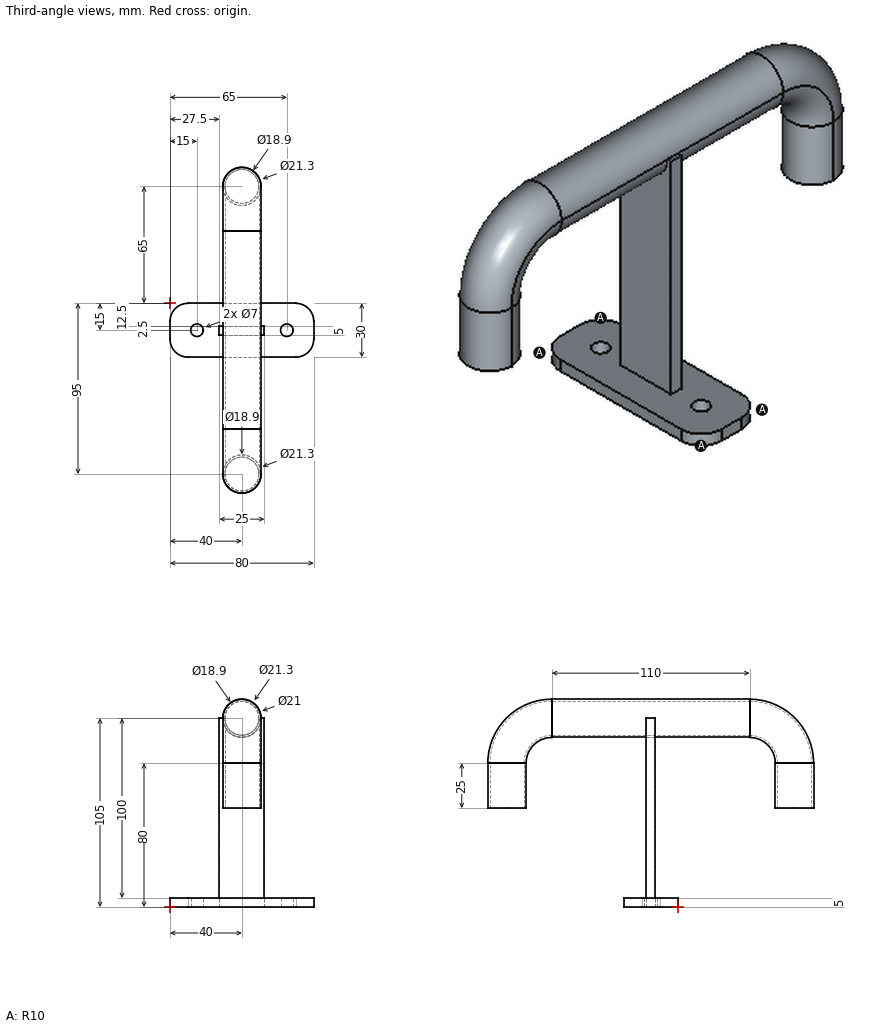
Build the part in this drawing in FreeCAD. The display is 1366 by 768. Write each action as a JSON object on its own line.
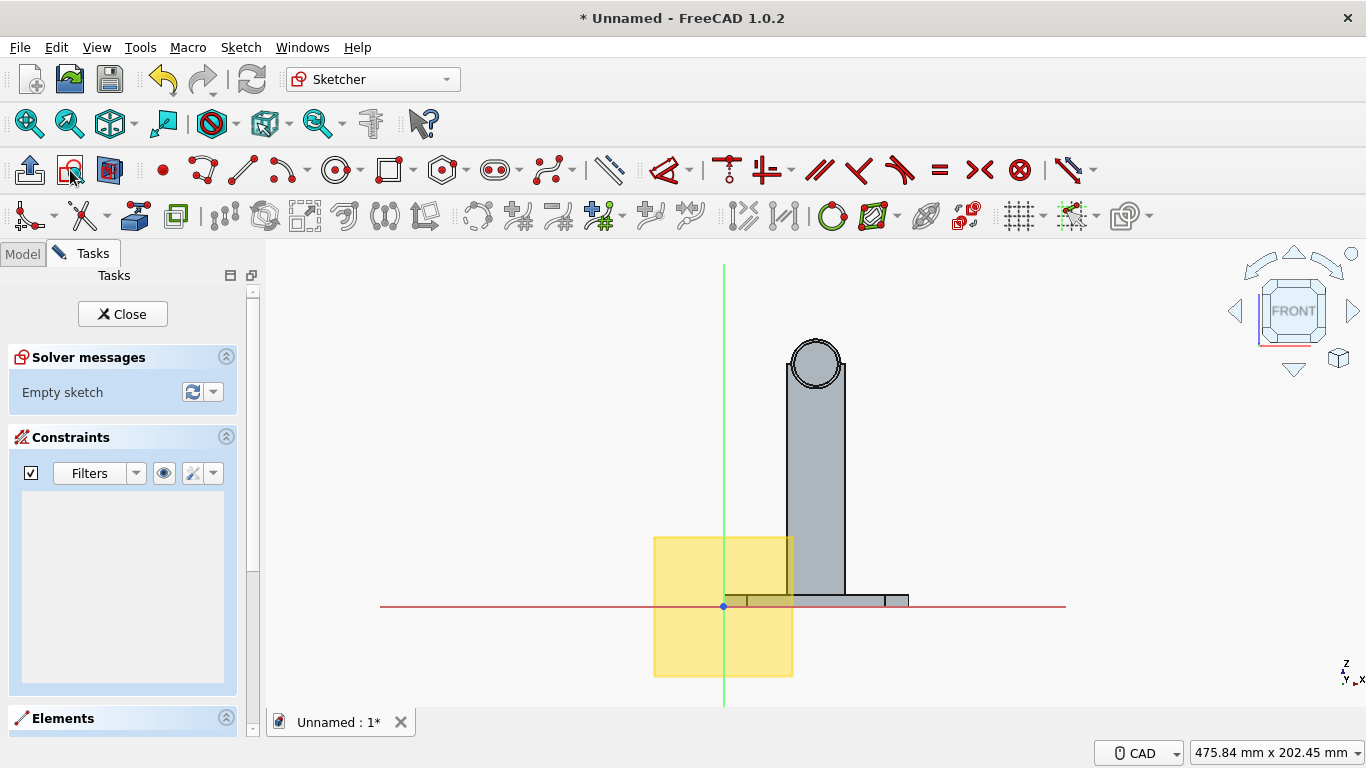
{"action": "scroll", "coordinate": [846, 341], "scroll_direction": "up", "scroll_amount": 6}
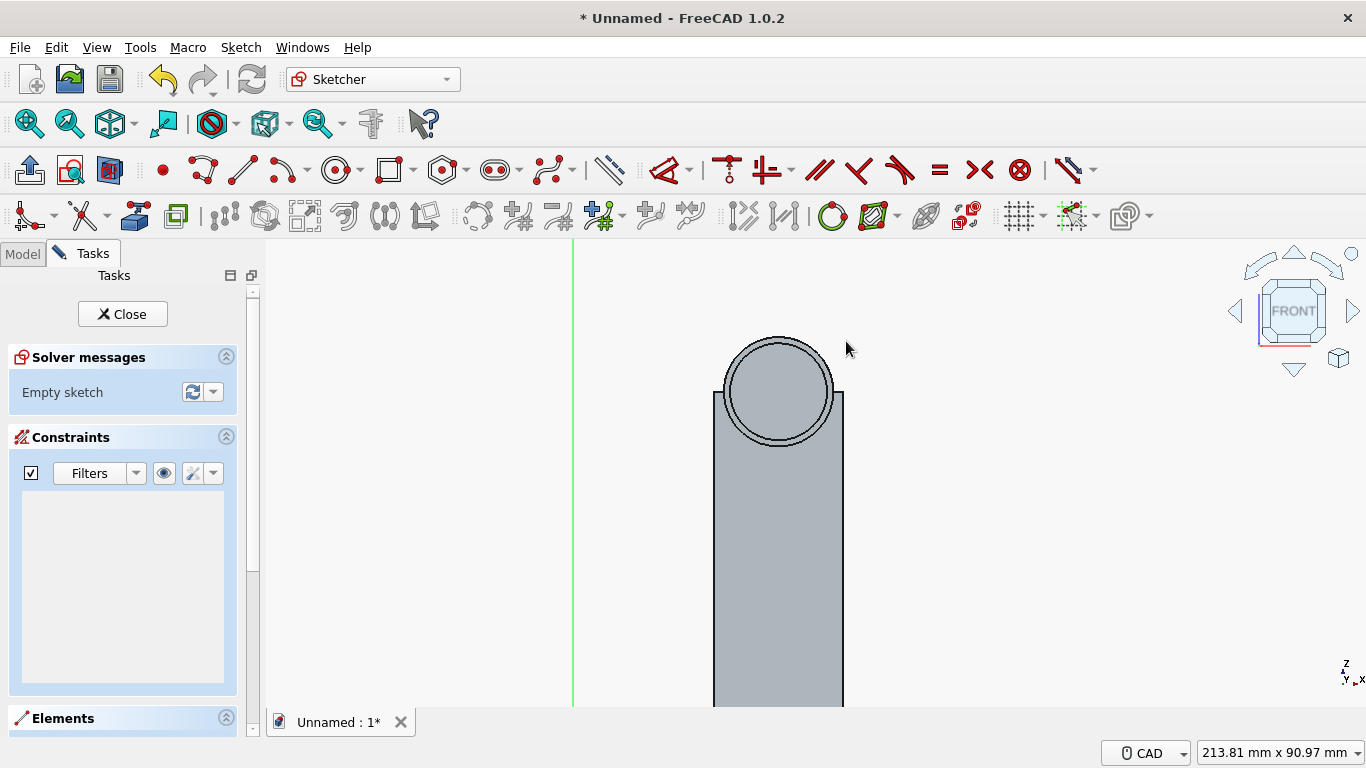
{"action": "left_click", "coordinate": [336, 170]}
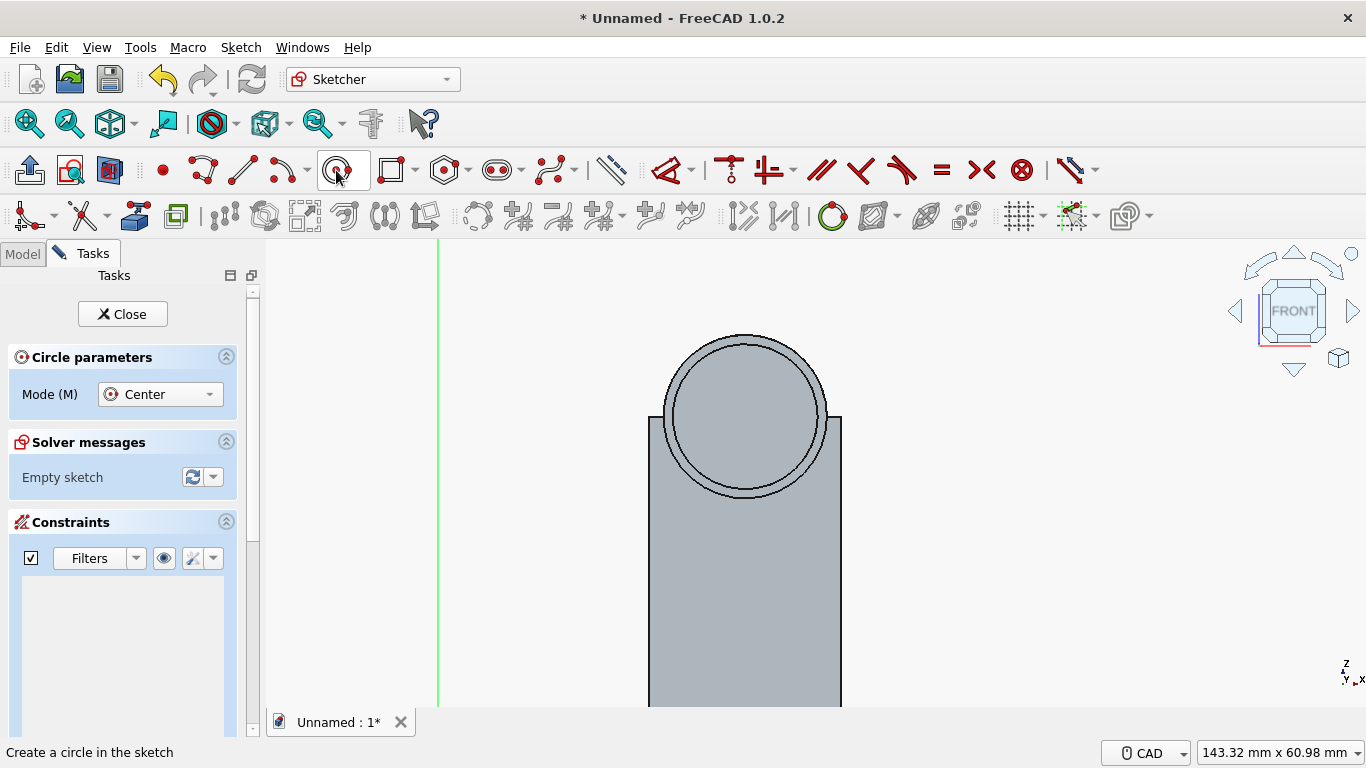
{"action": "left_click", "coordinate": [745, 417]}
{"action": "mouse_move", "coordinate": [803, 359]}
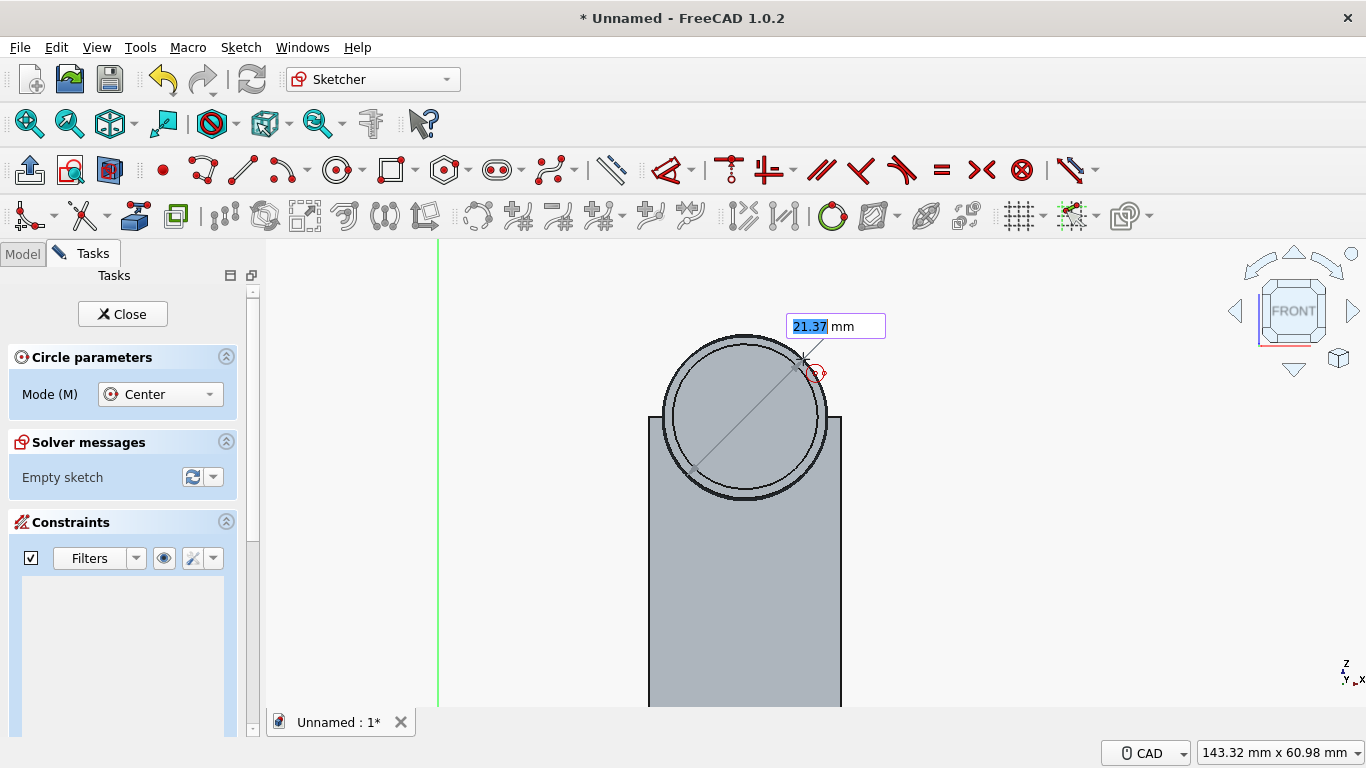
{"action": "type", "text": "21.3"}
{"action": "key", "text": "Return"}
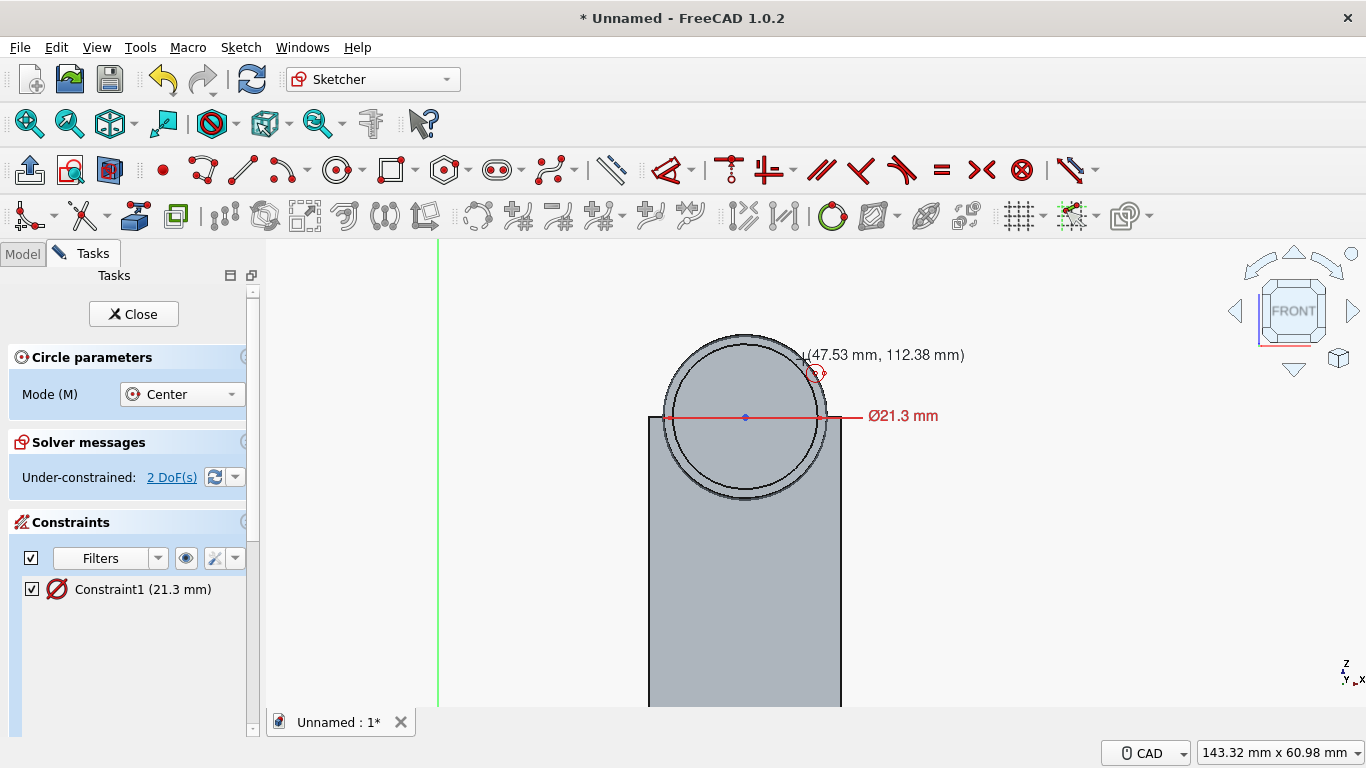
{"action": "left_click", "coordinate": [745, 418]}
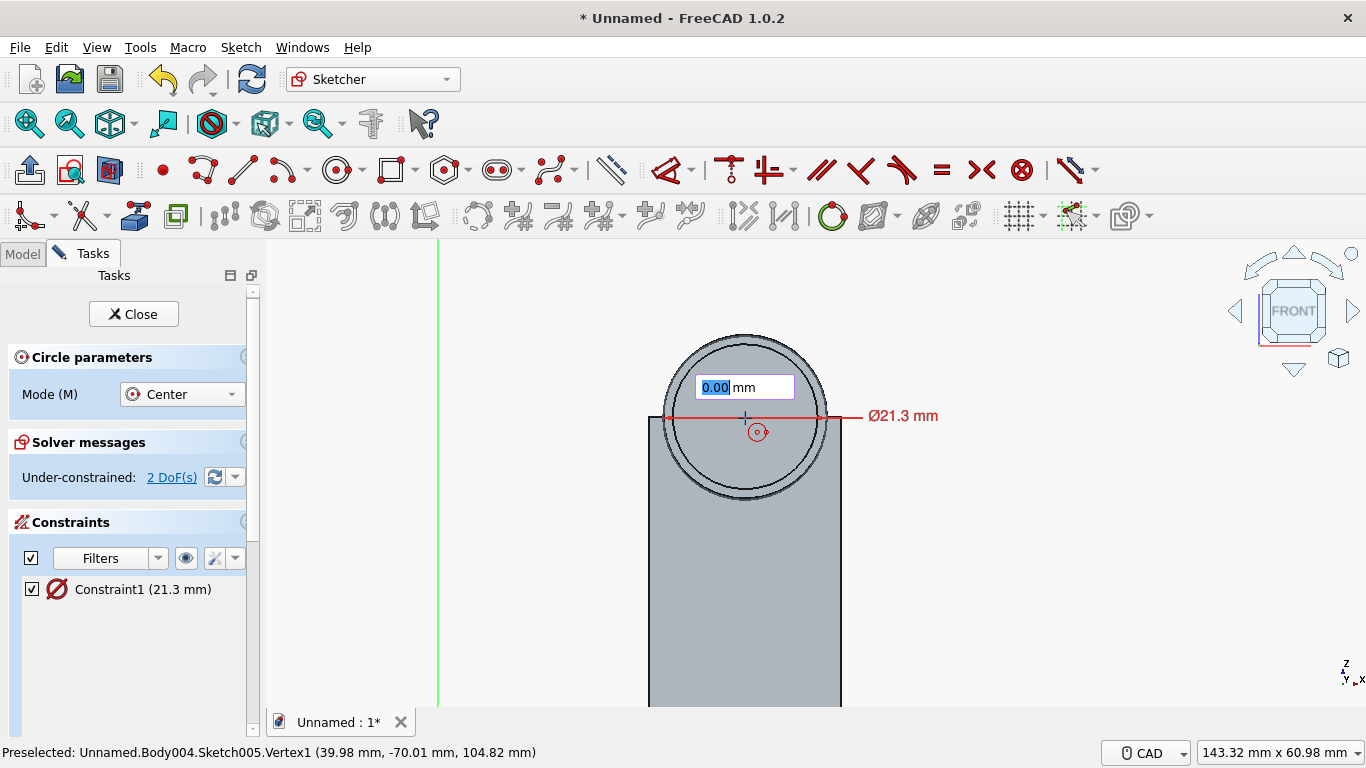
{"action": "scroll", "coordinate": [796, 468], "scroll_direction": "up", "scroll_amount": 3}
{"action": "mouse_move", "coordinate": [796, 467]}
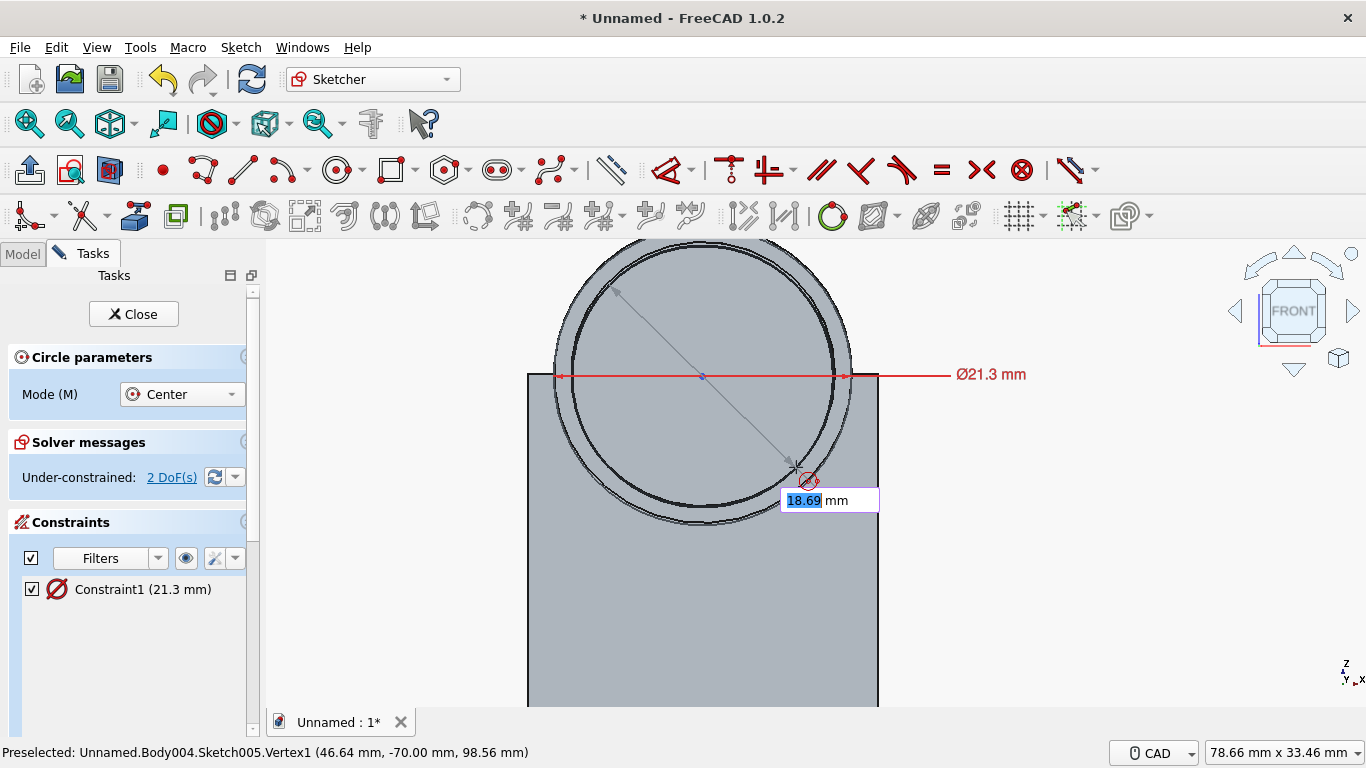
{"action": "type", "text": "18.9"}
{"action": "key", "text": "Return"}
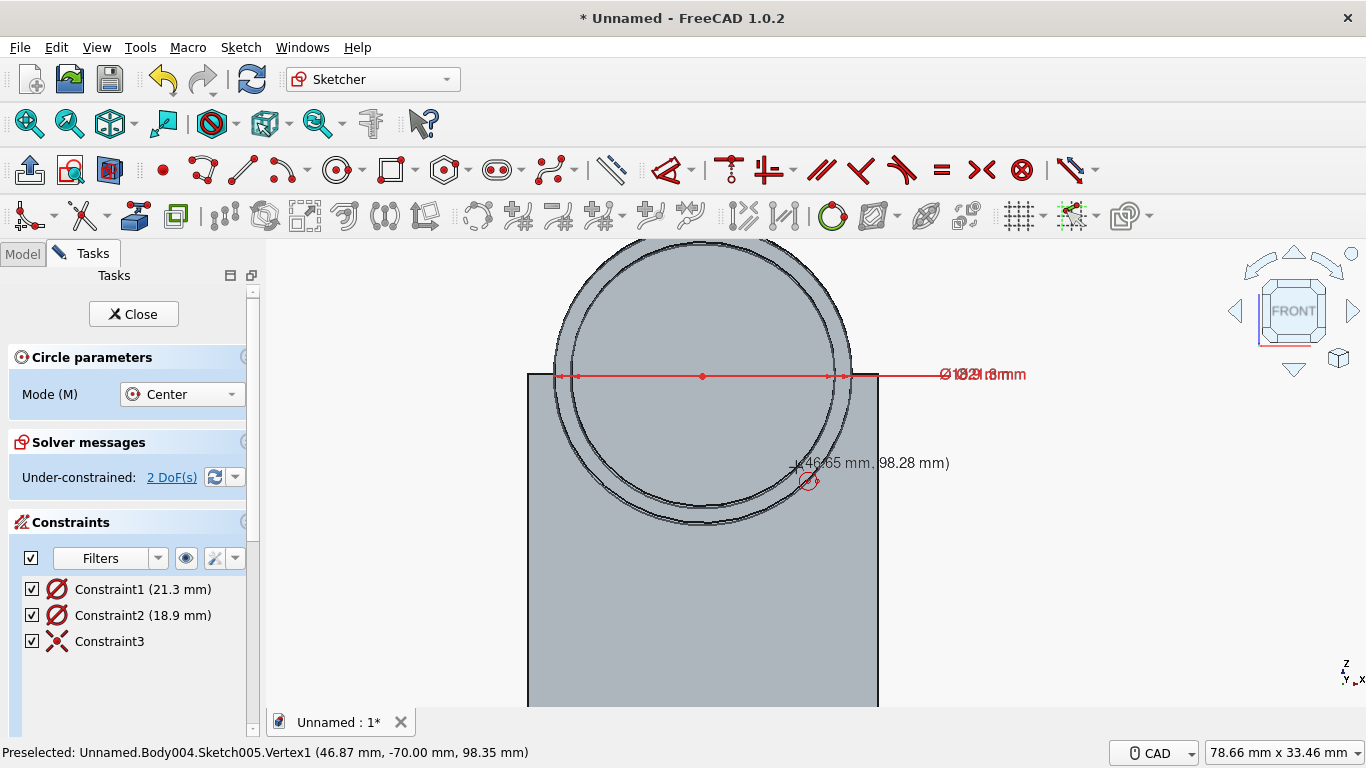
{"action": "left_click", "coordinate": [244, 170]}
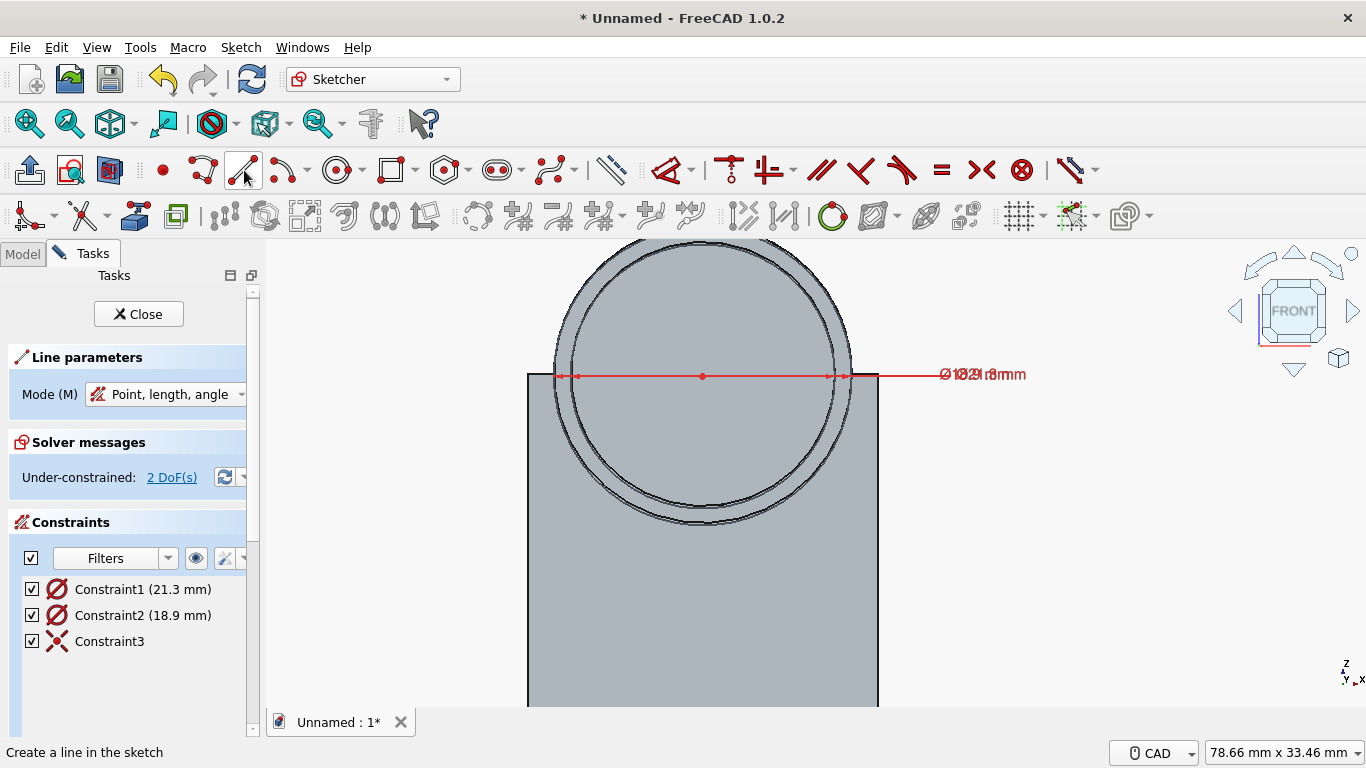
{"action": "scroll", "coordinate": [802, 471], "scroll_direction": "down", "scroll_amount": 3}